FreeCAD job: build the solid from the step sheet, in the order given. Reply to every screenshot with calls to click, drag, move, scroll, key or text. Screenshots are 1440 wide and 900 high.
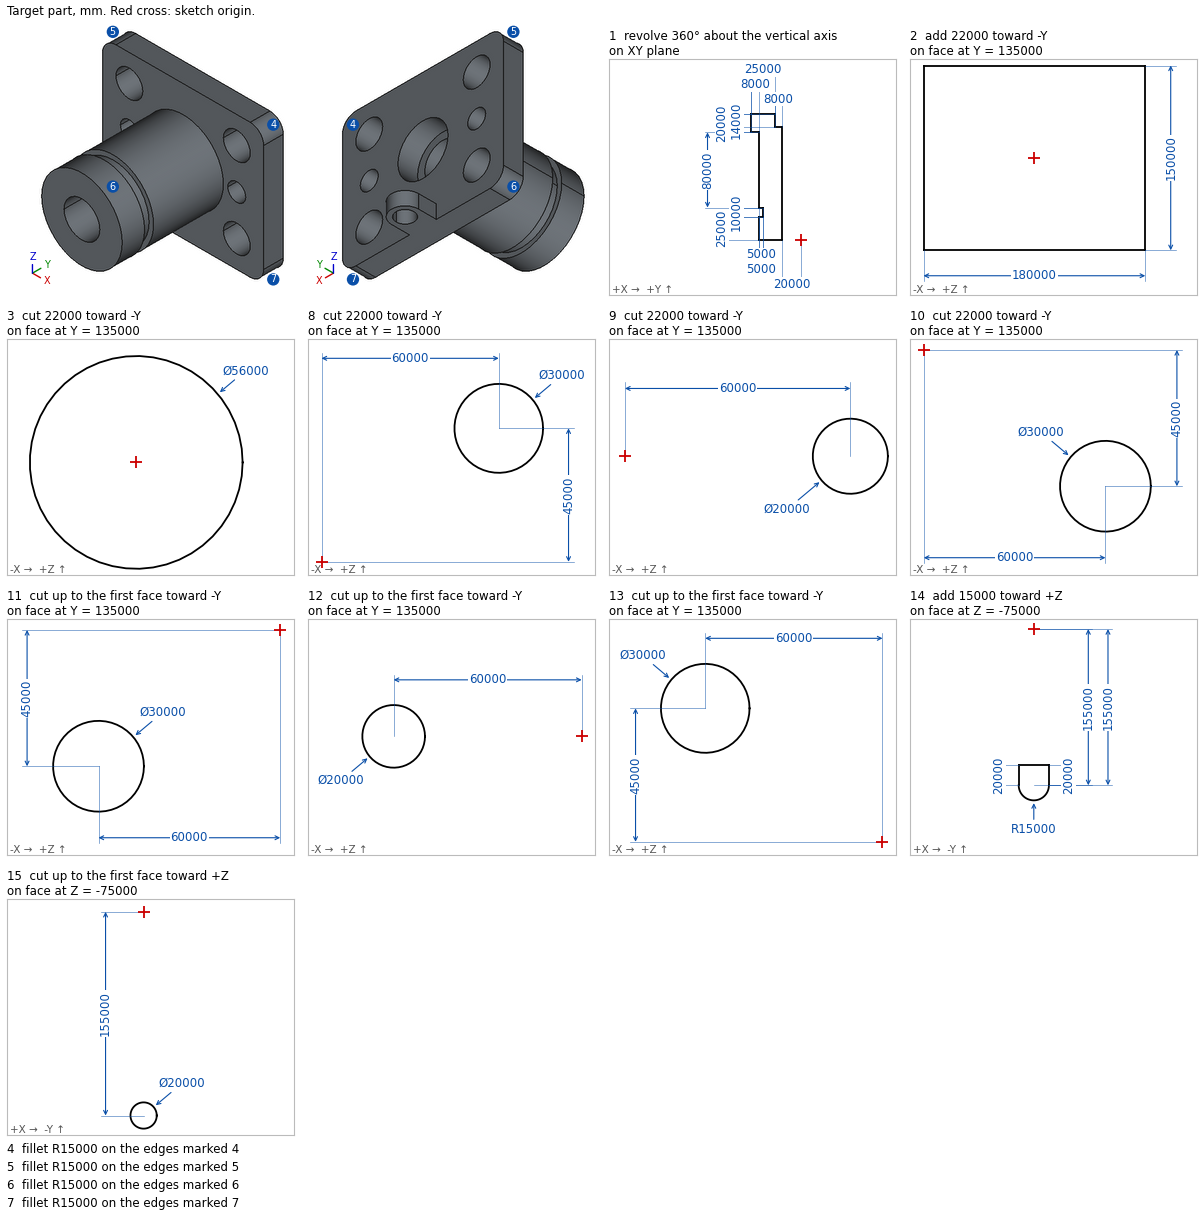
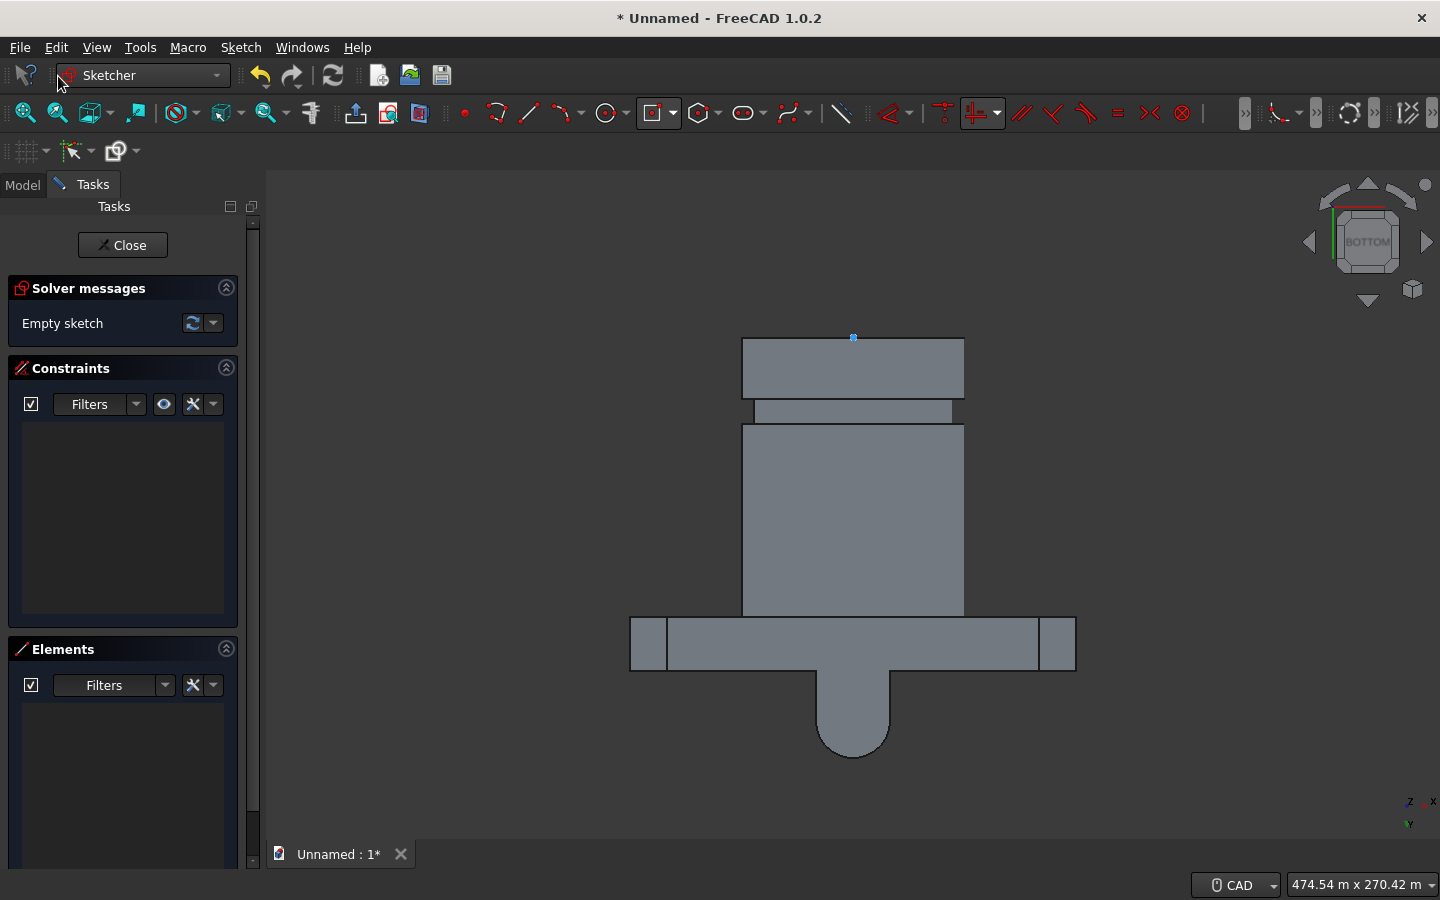
scroll(862, 748, up, 11)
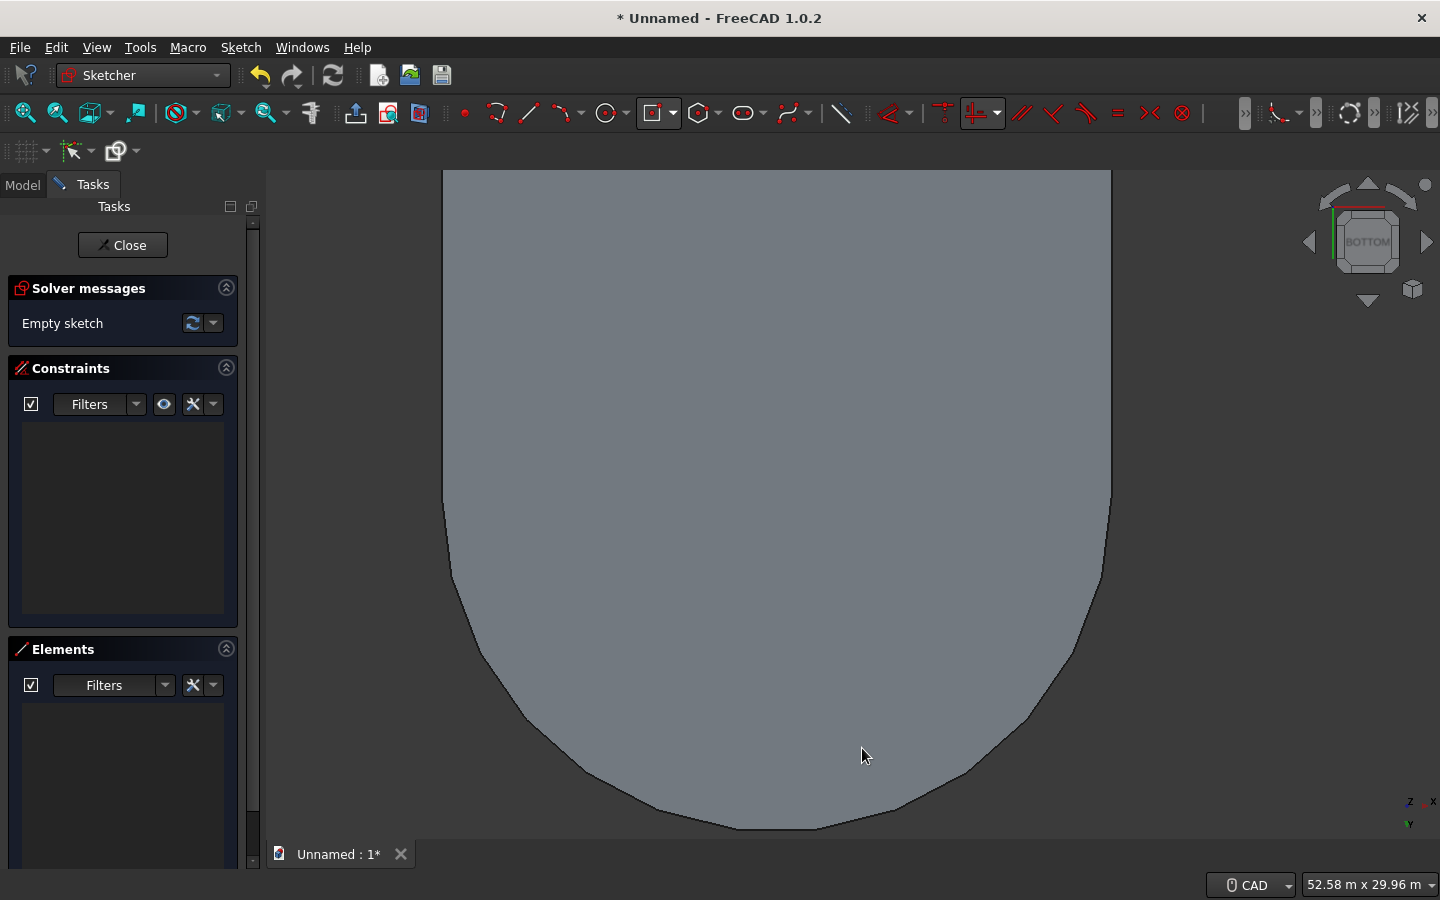
click(606, 114)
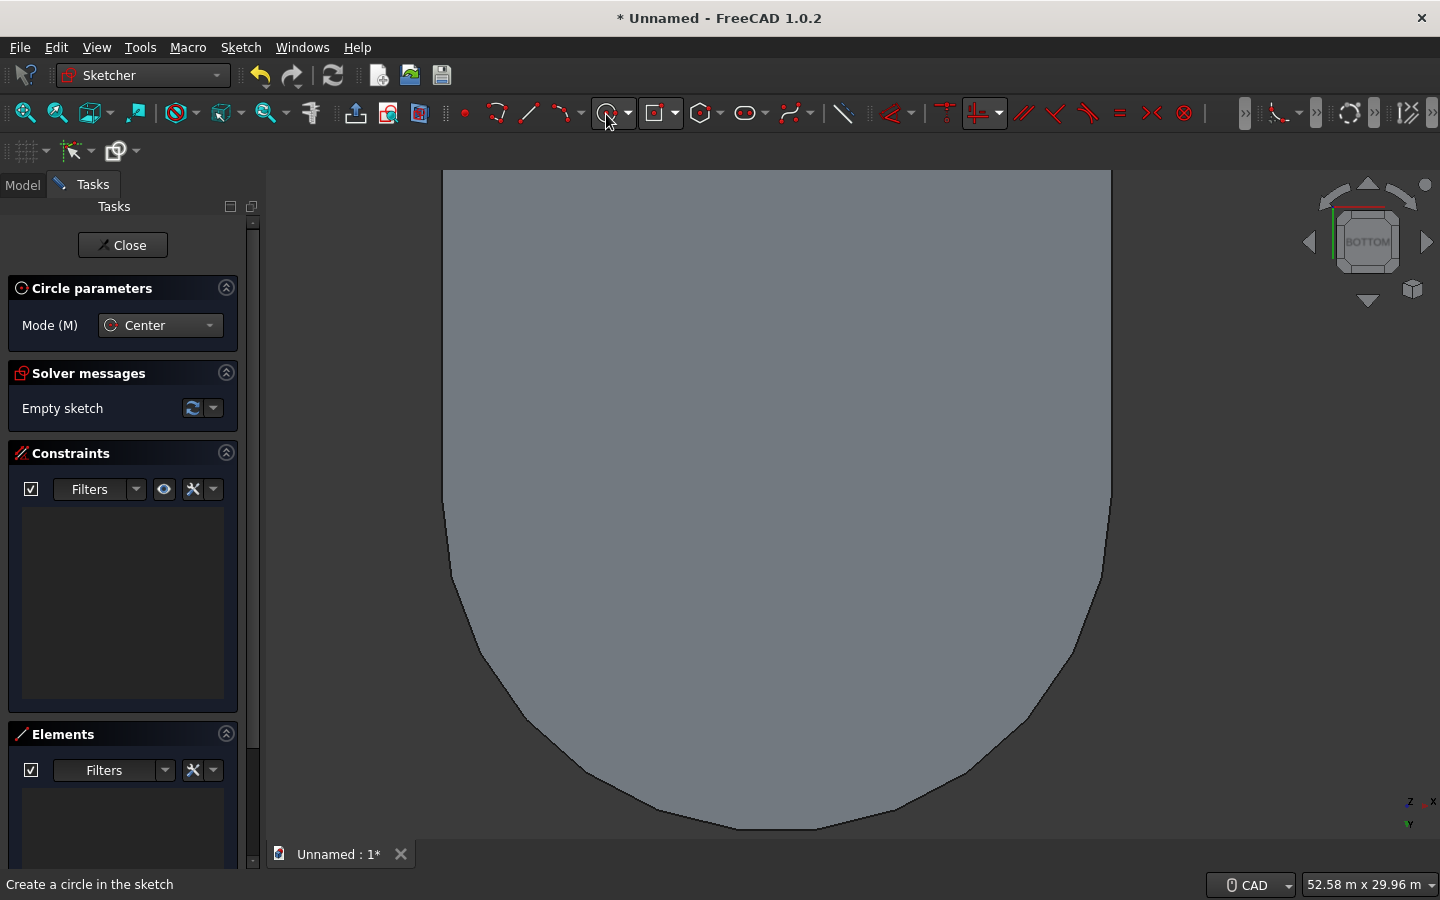
click(777, 497)
click(935, 339)
key(Escape)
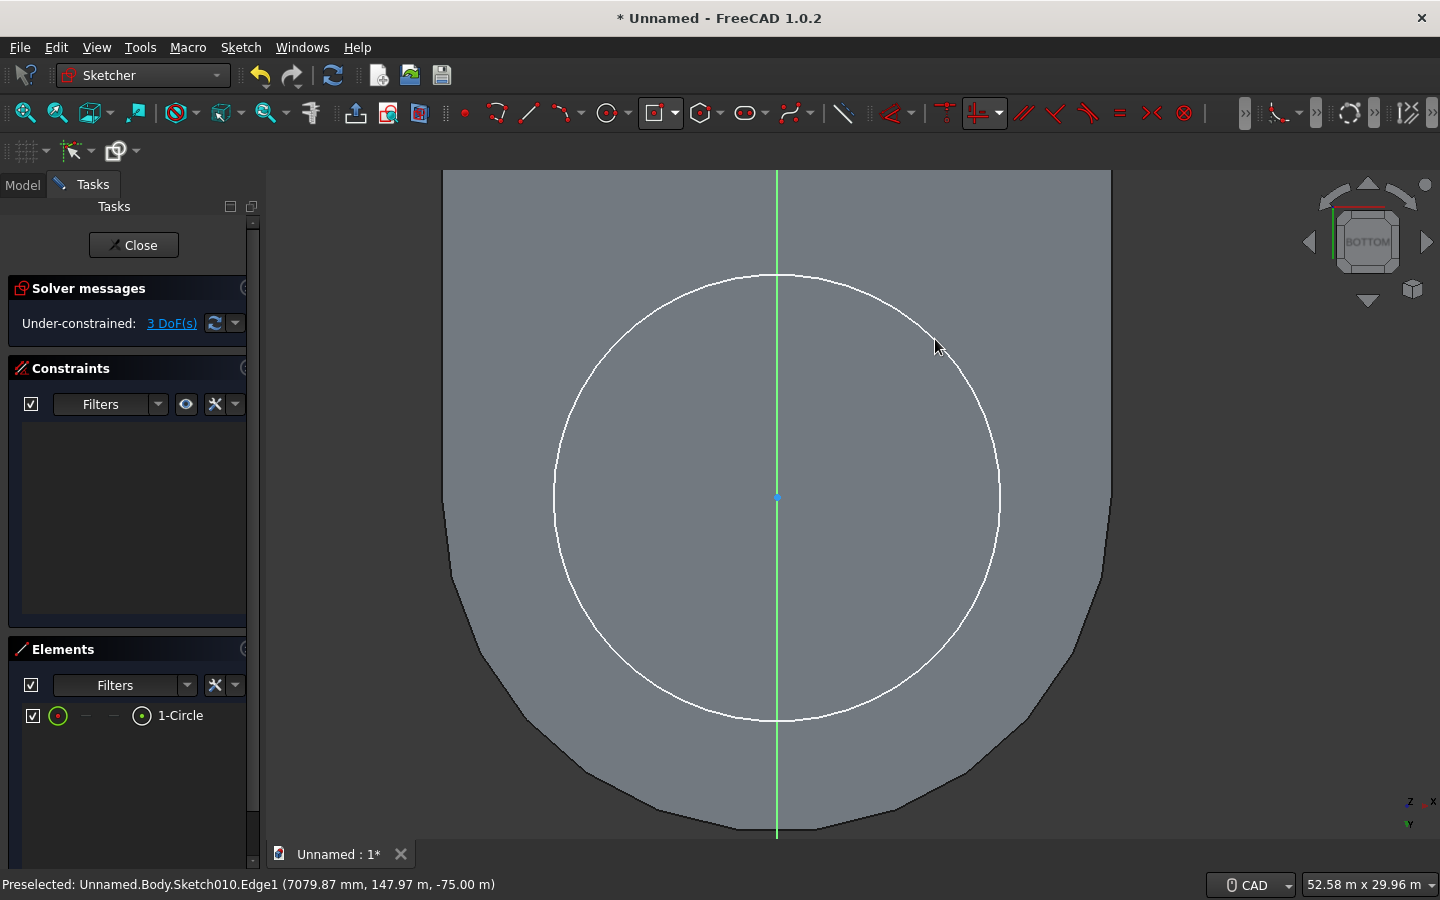
click(777, 498)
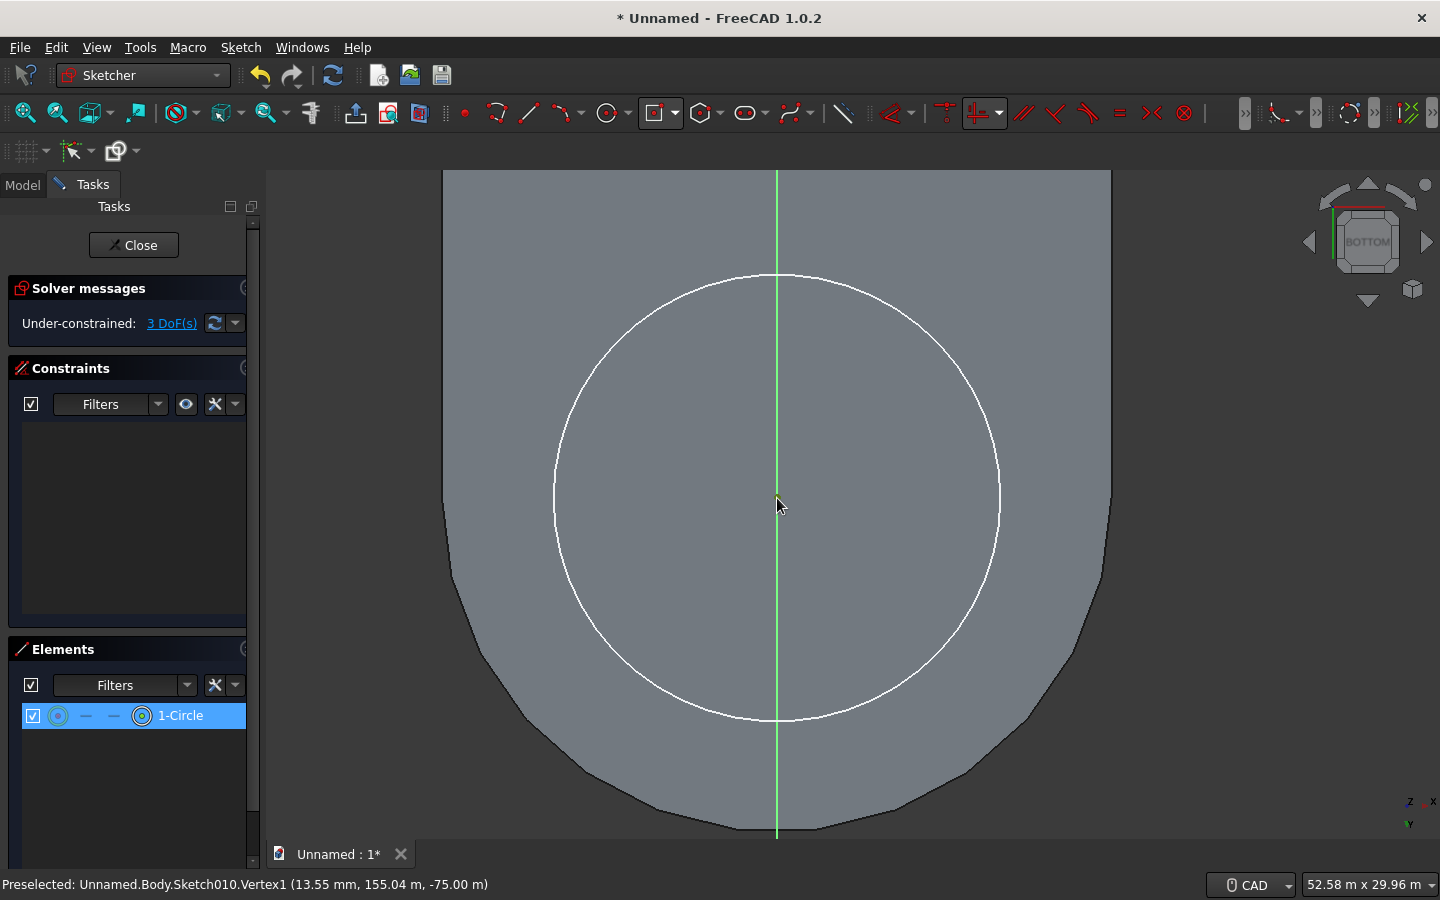
click(777, 767)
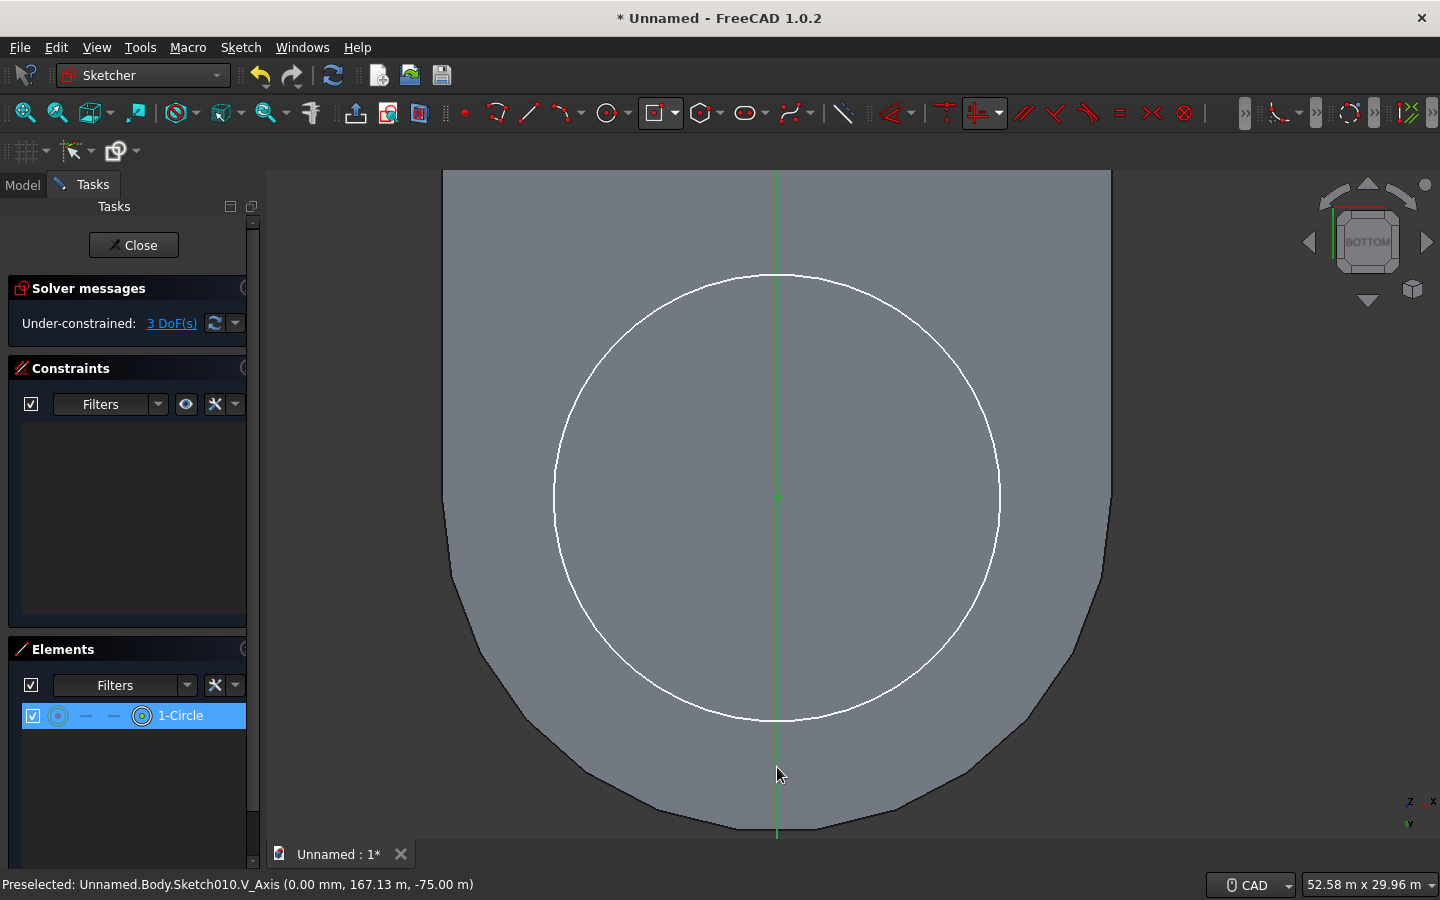
click(946, 114)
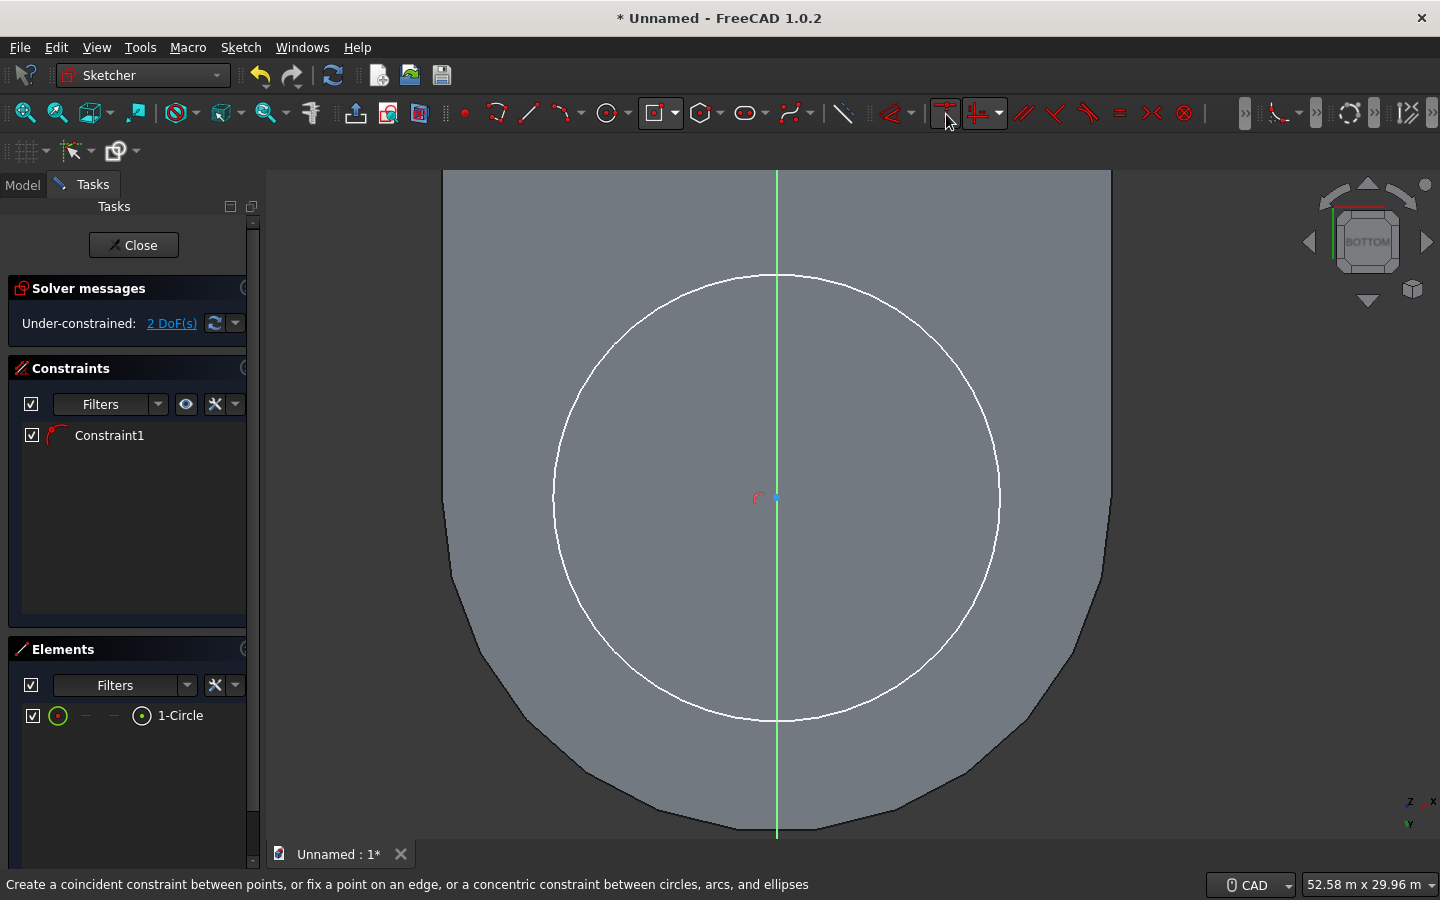
click(890, 114)